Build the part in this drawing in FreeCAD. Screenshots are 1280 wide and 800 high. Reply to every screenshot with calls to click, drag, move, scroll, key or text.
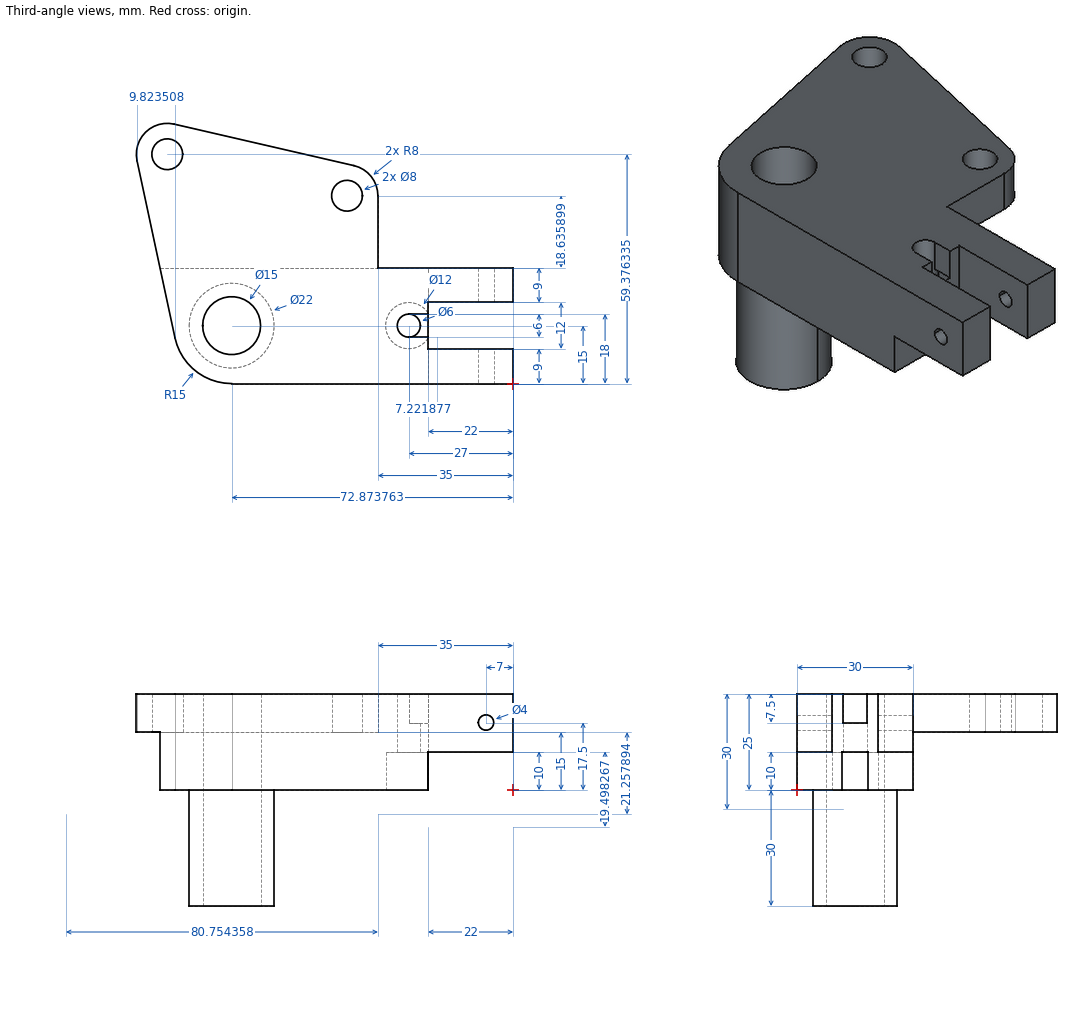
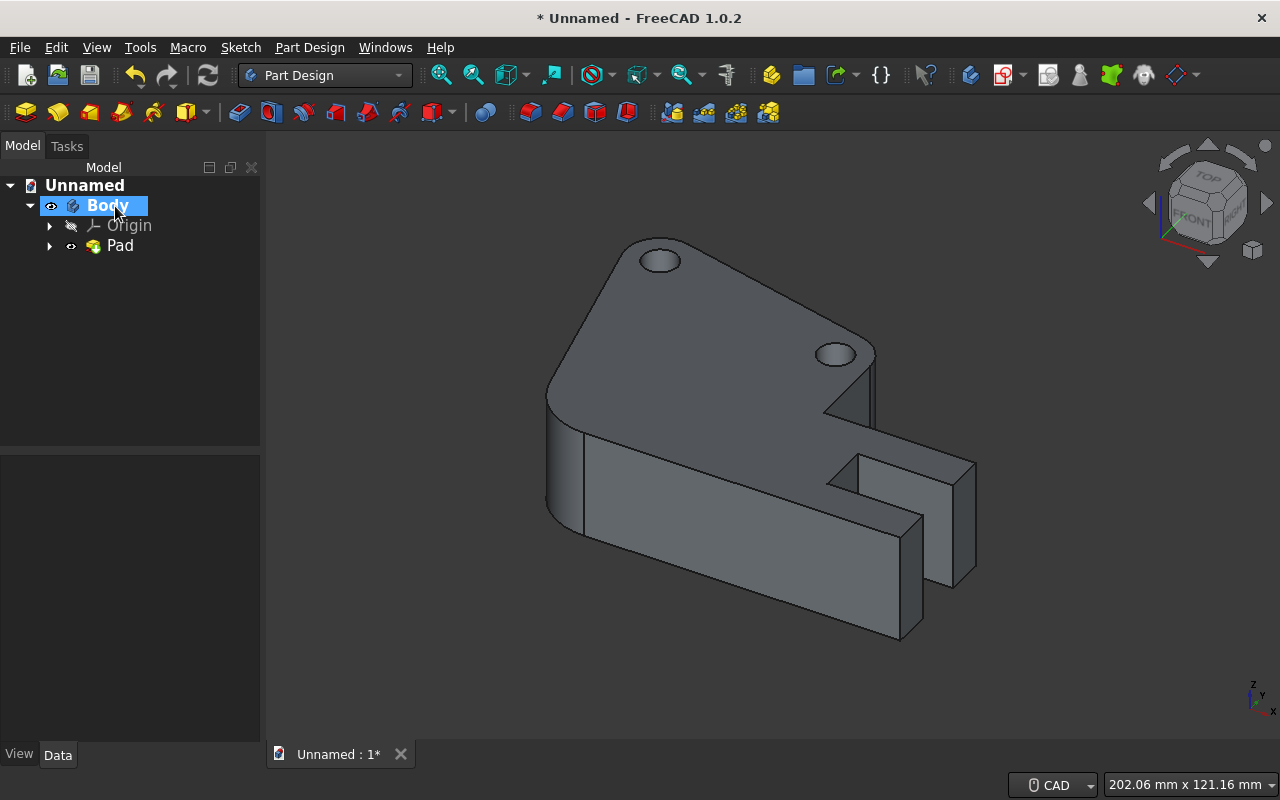
key(4)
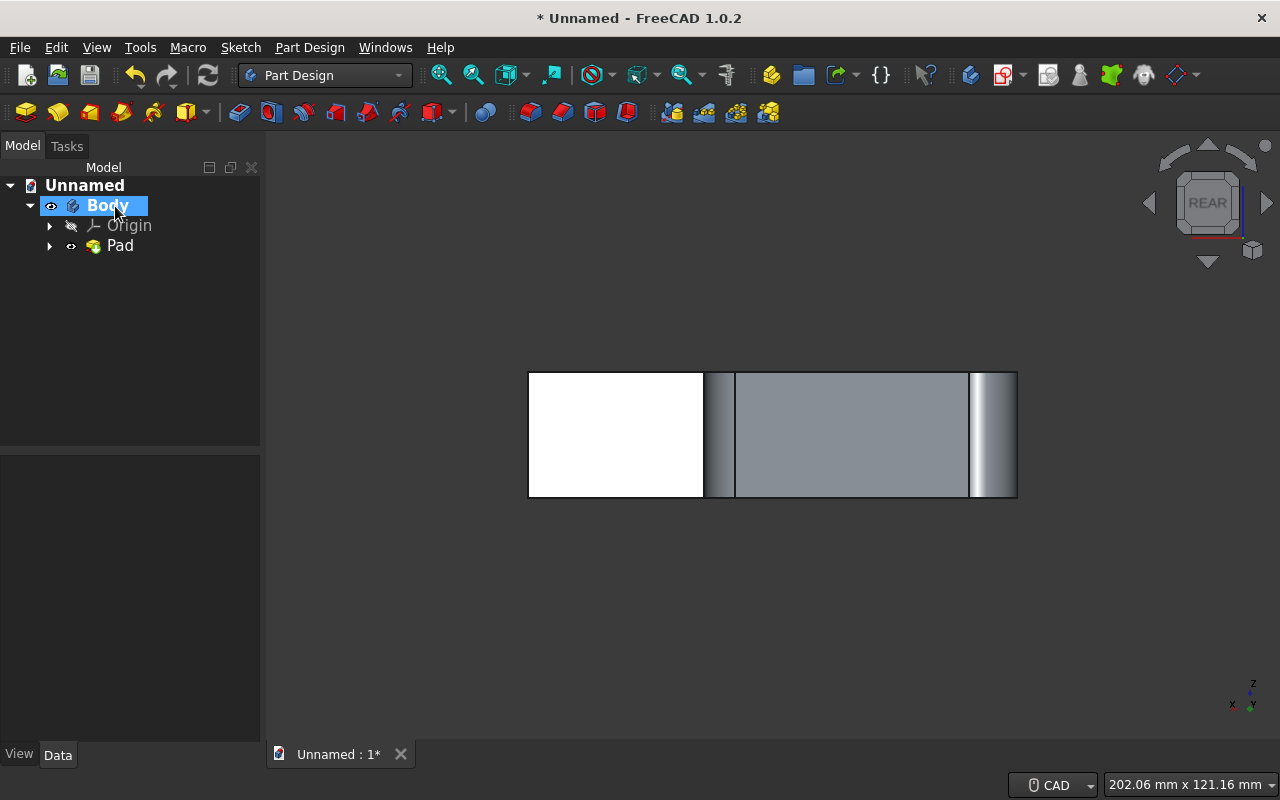
click(591, 434)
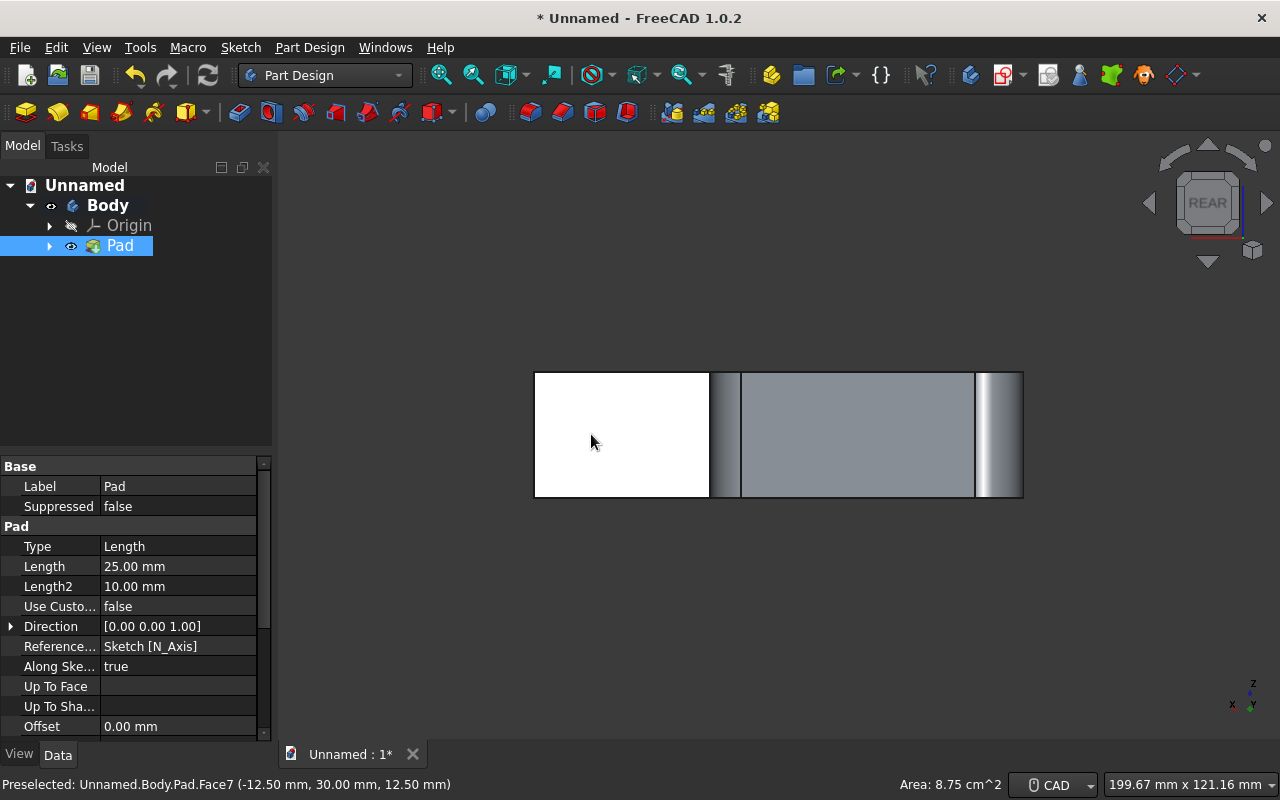
click(1004, 76)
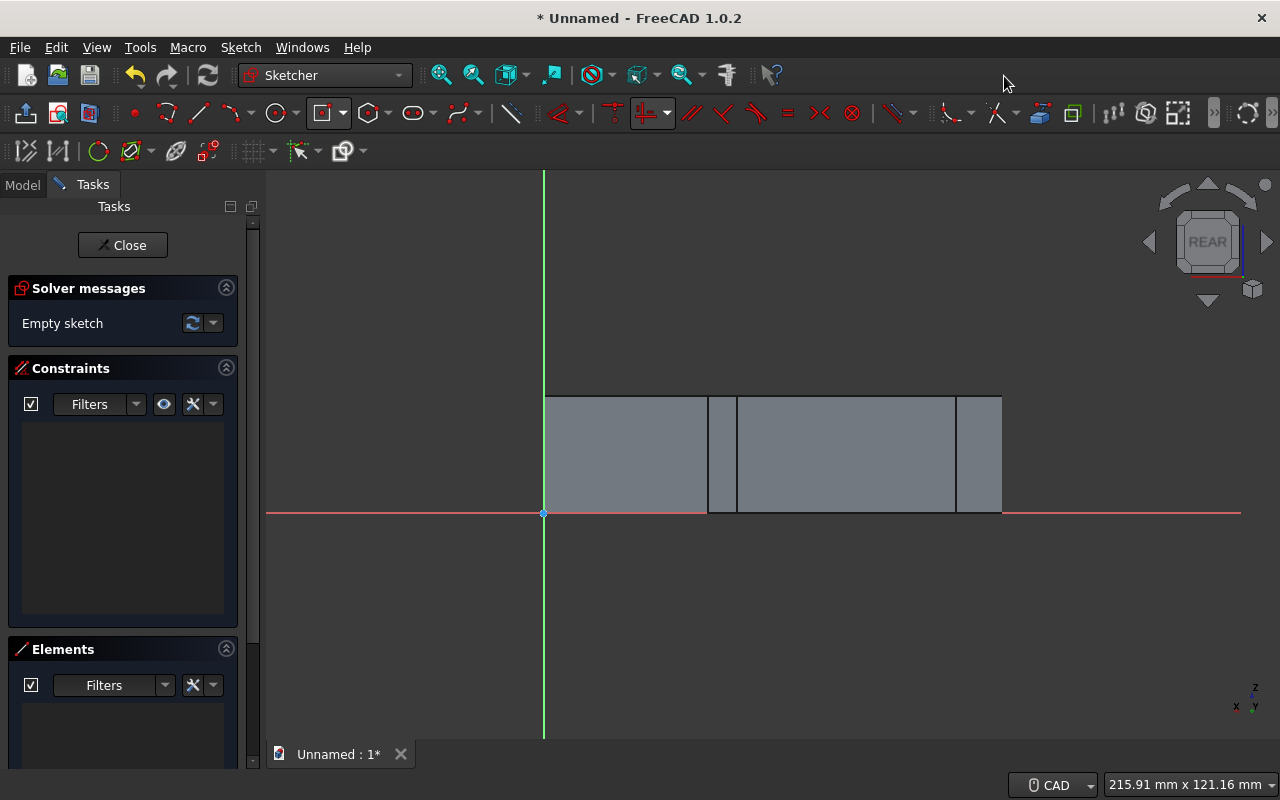
click(90, 114)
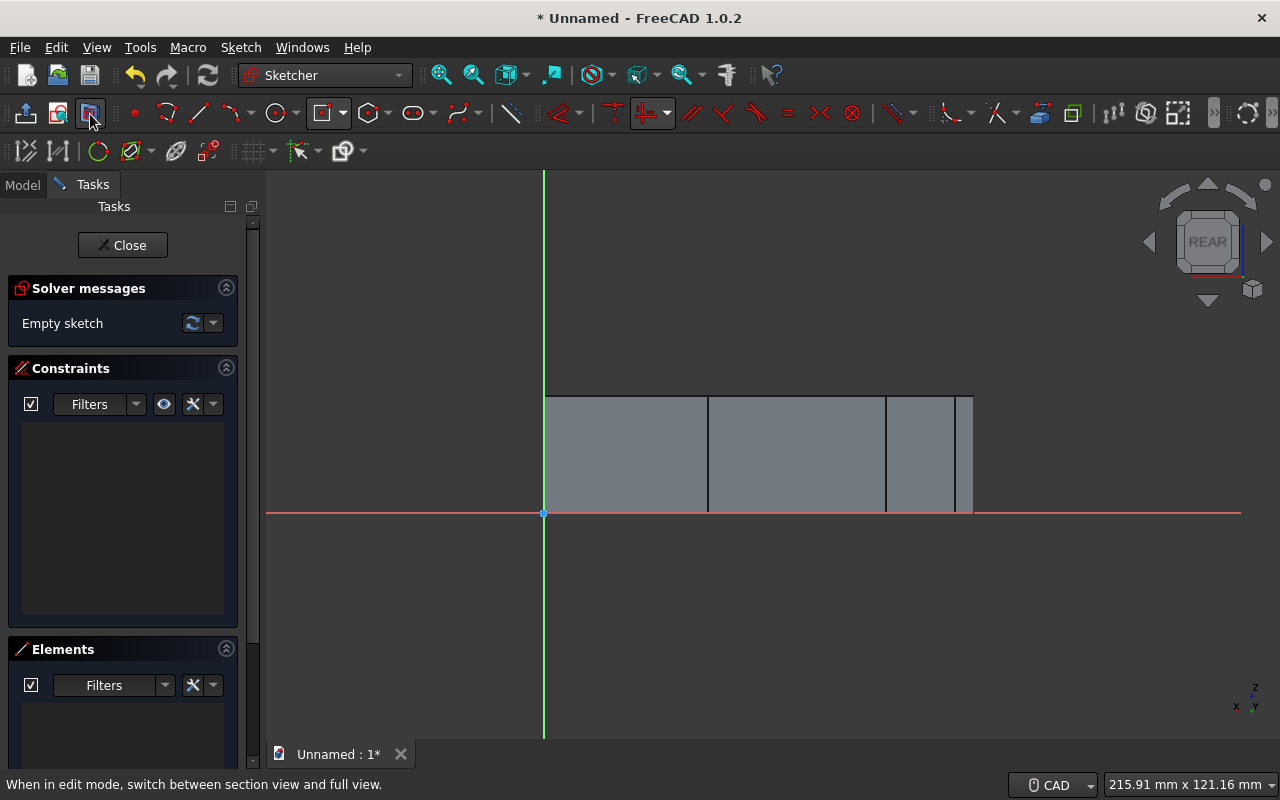
click(346, 114)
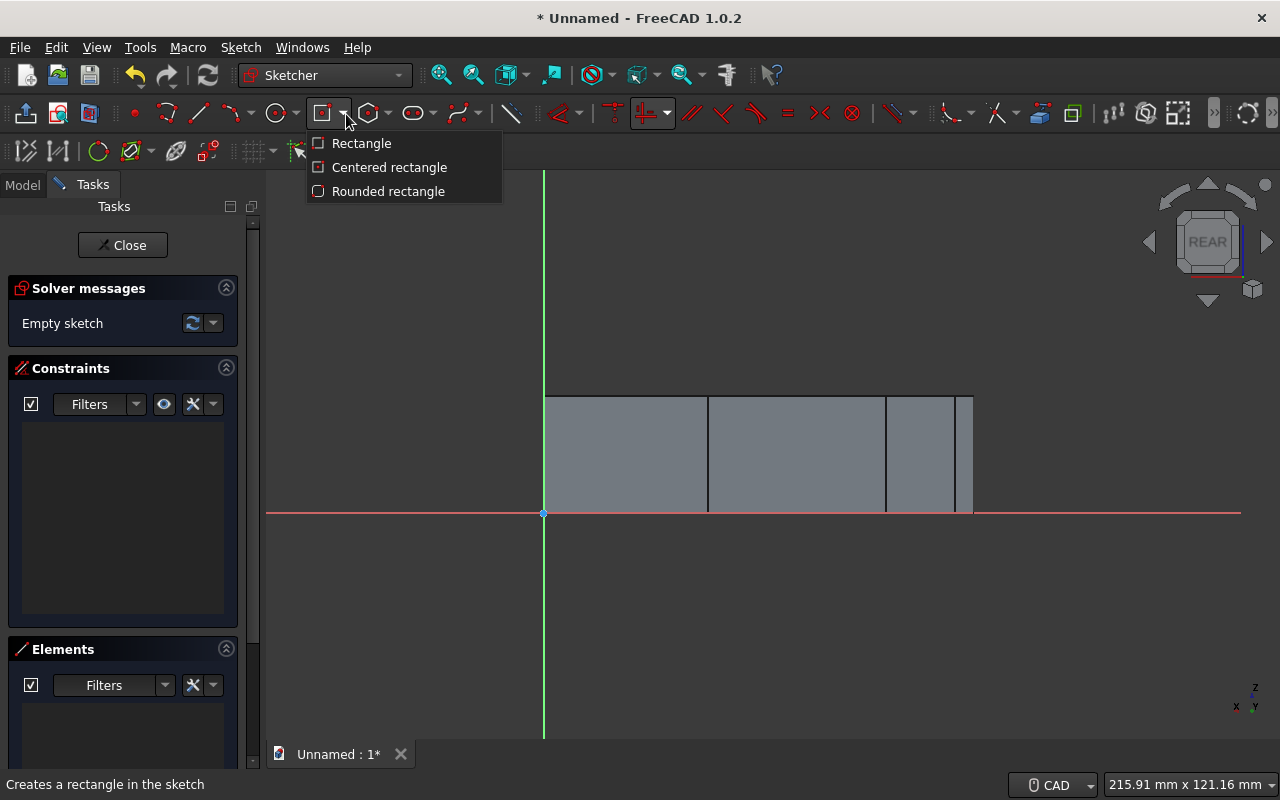
click(404, 143)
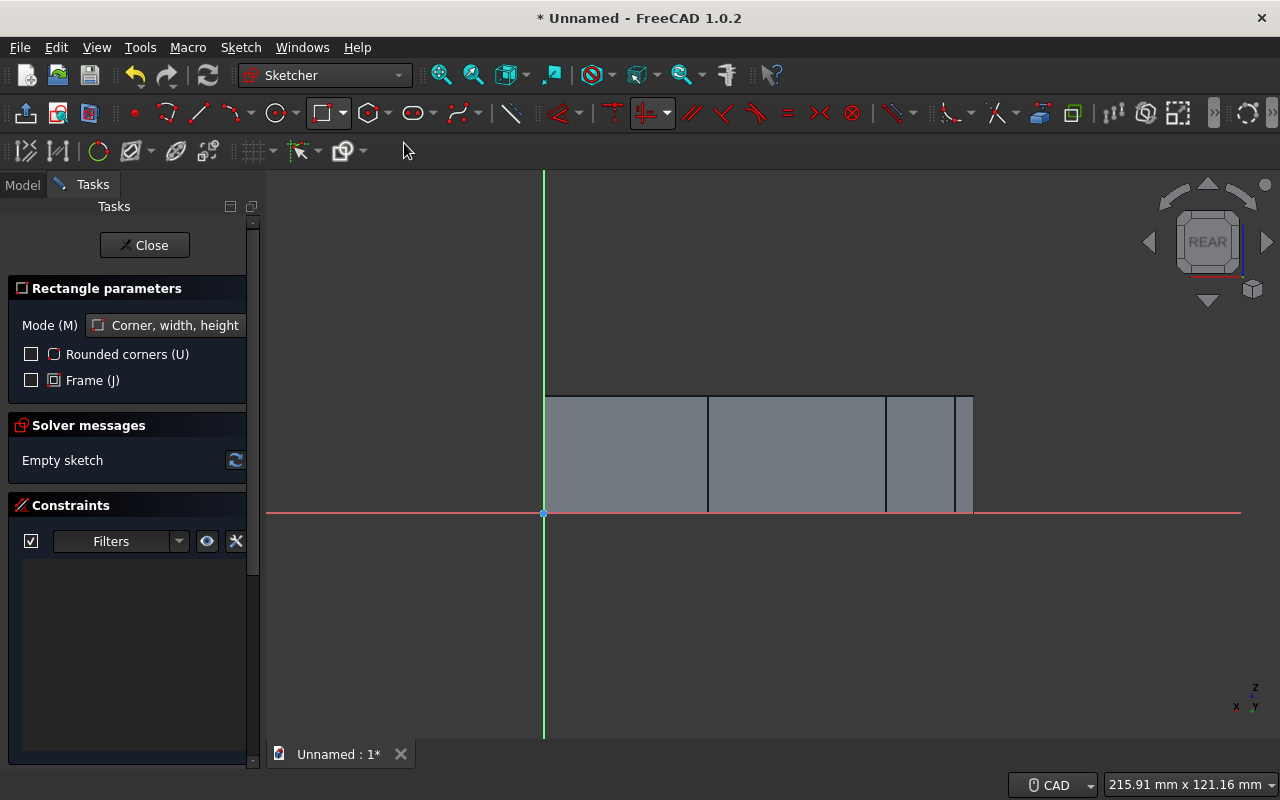
click(708, 443)
click(1088, 543)
key(Escape)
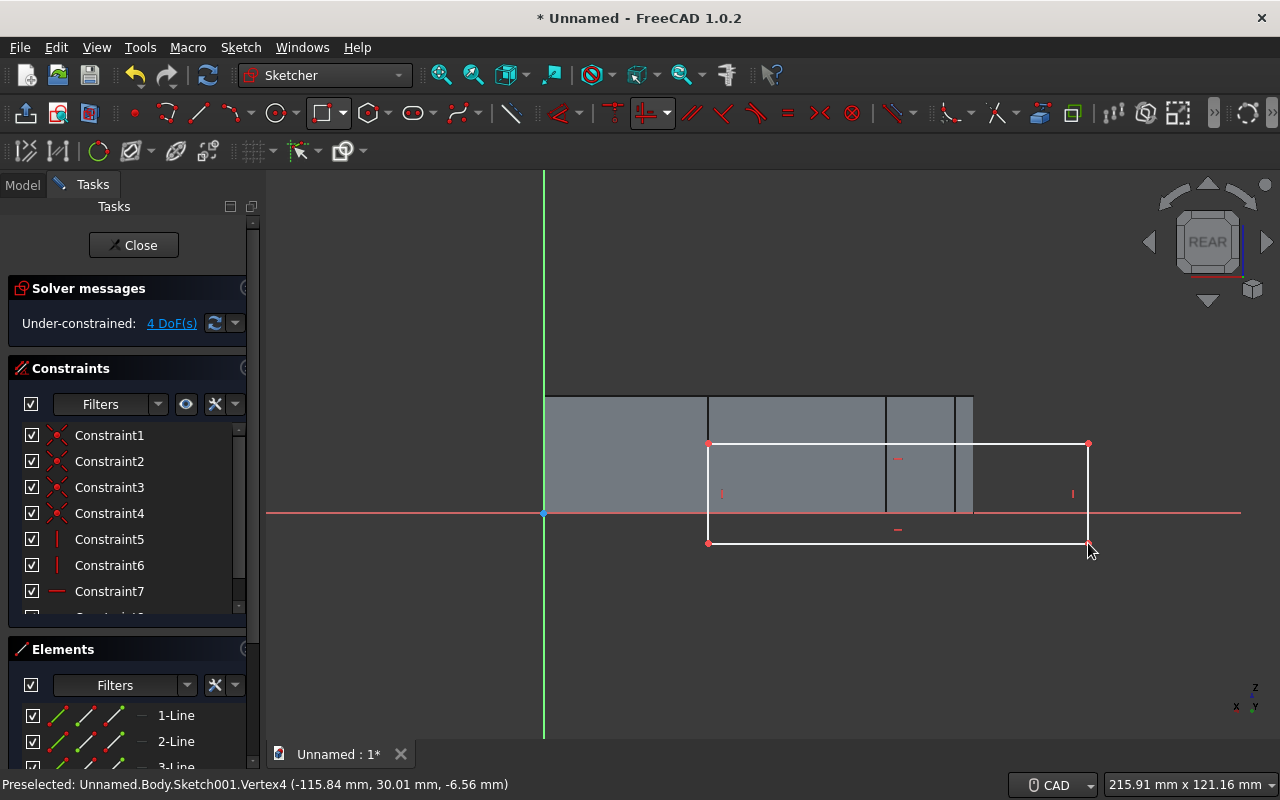
click(558, 114)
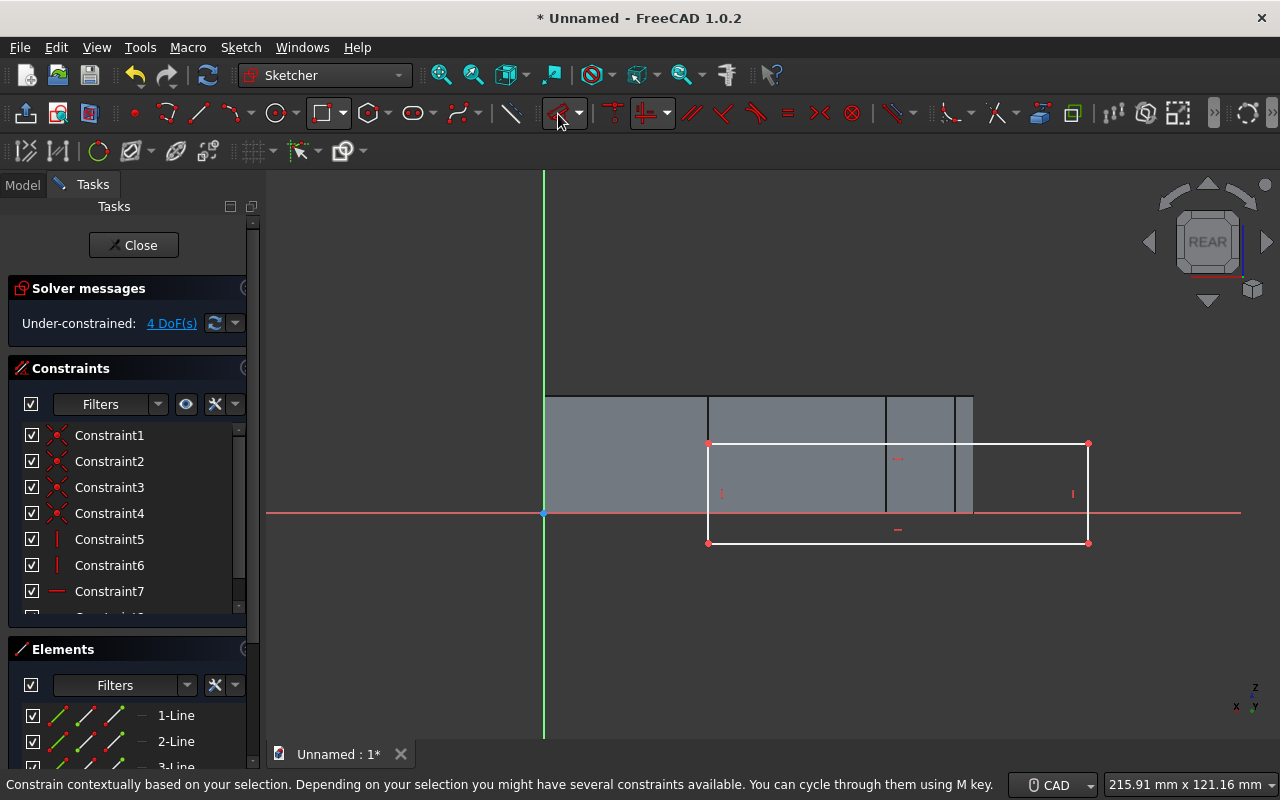
click(708, 444)
click(626, 410)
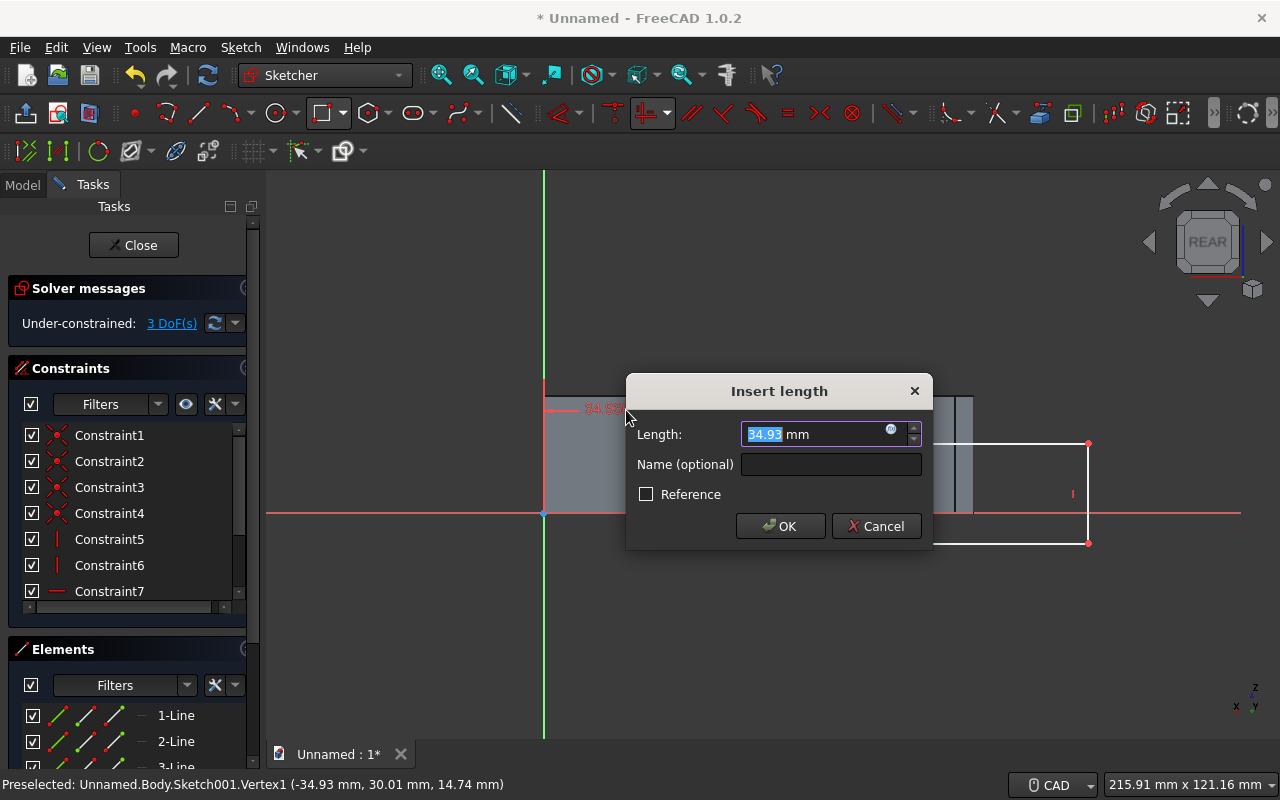
text(35)
key(Return)